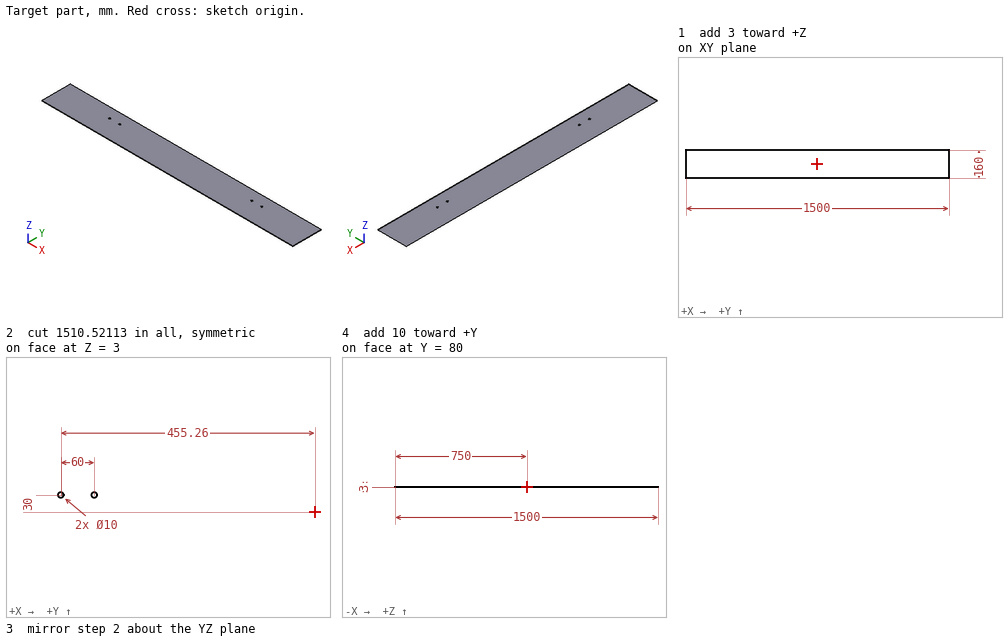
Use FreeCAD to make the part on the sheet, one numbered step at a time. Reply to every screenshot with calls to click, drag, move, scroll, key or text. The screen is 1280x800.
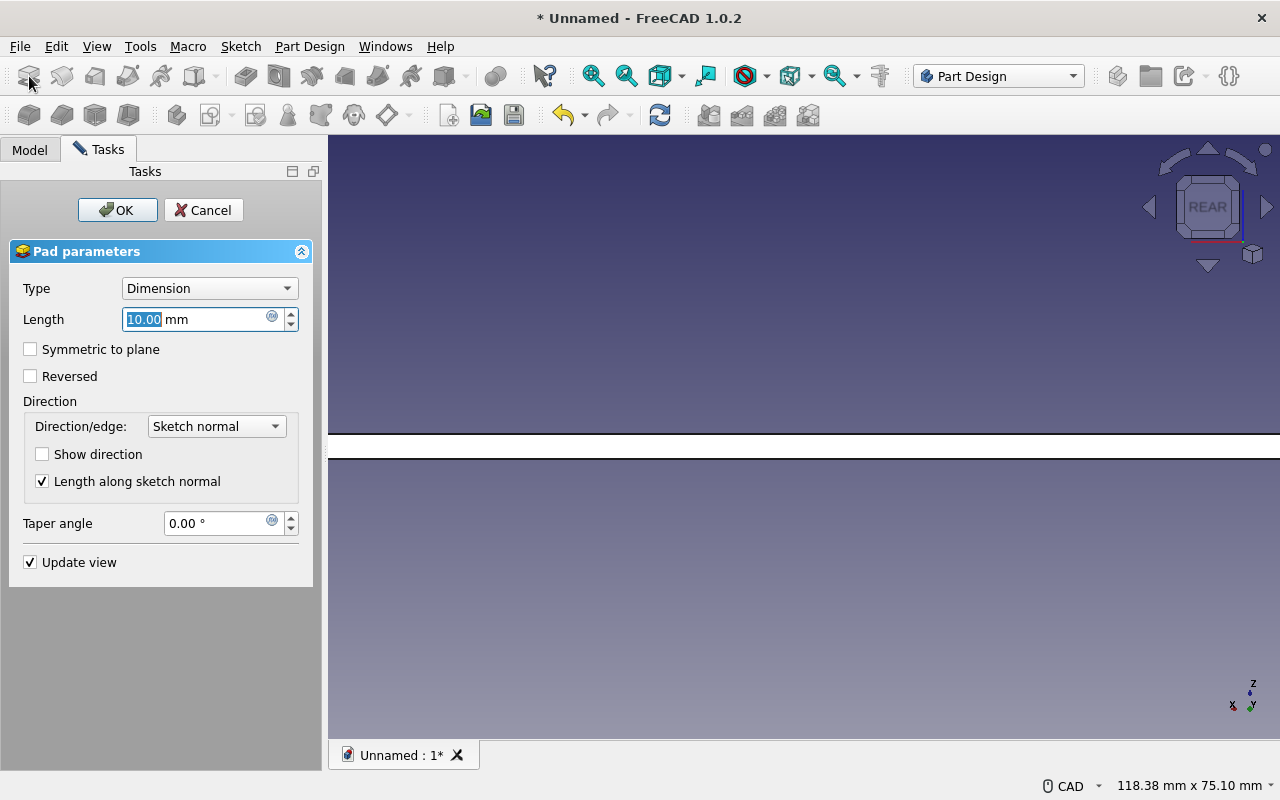
text(10)
key(Tab)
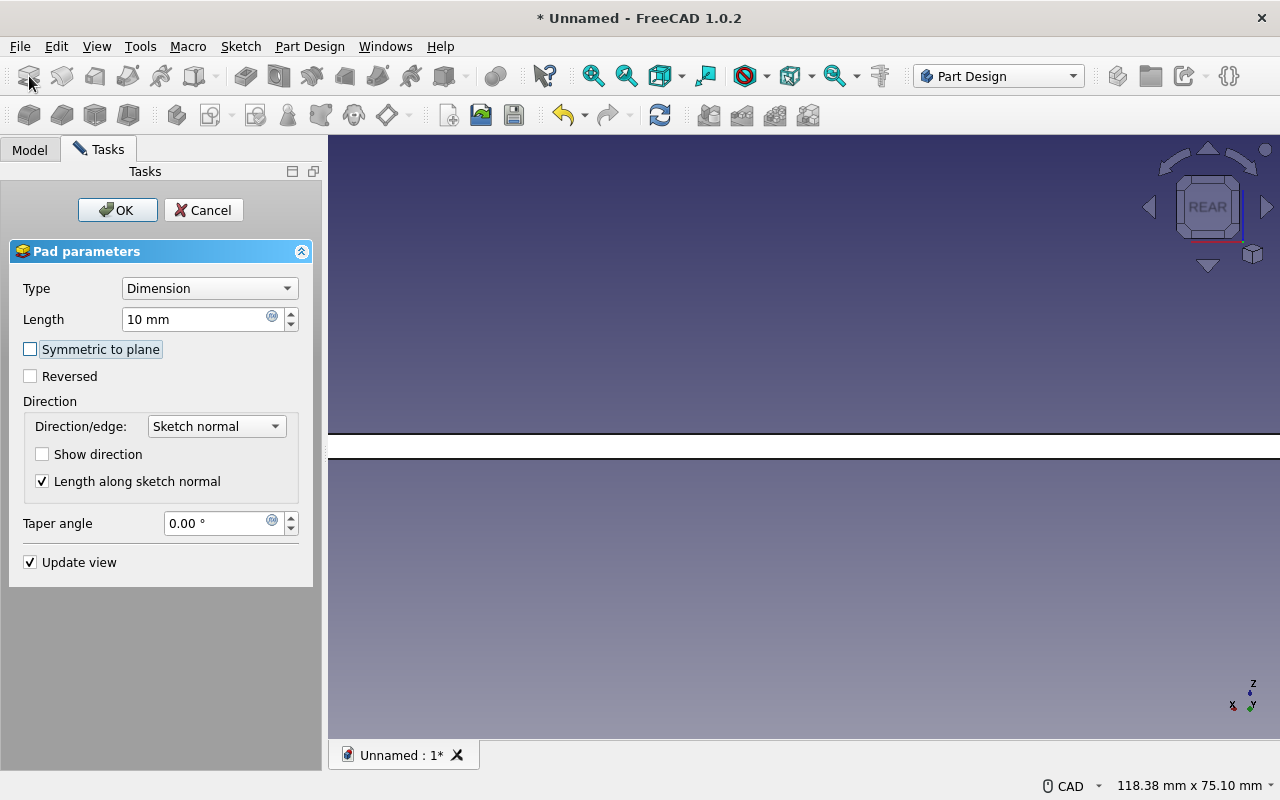
click(118, 210)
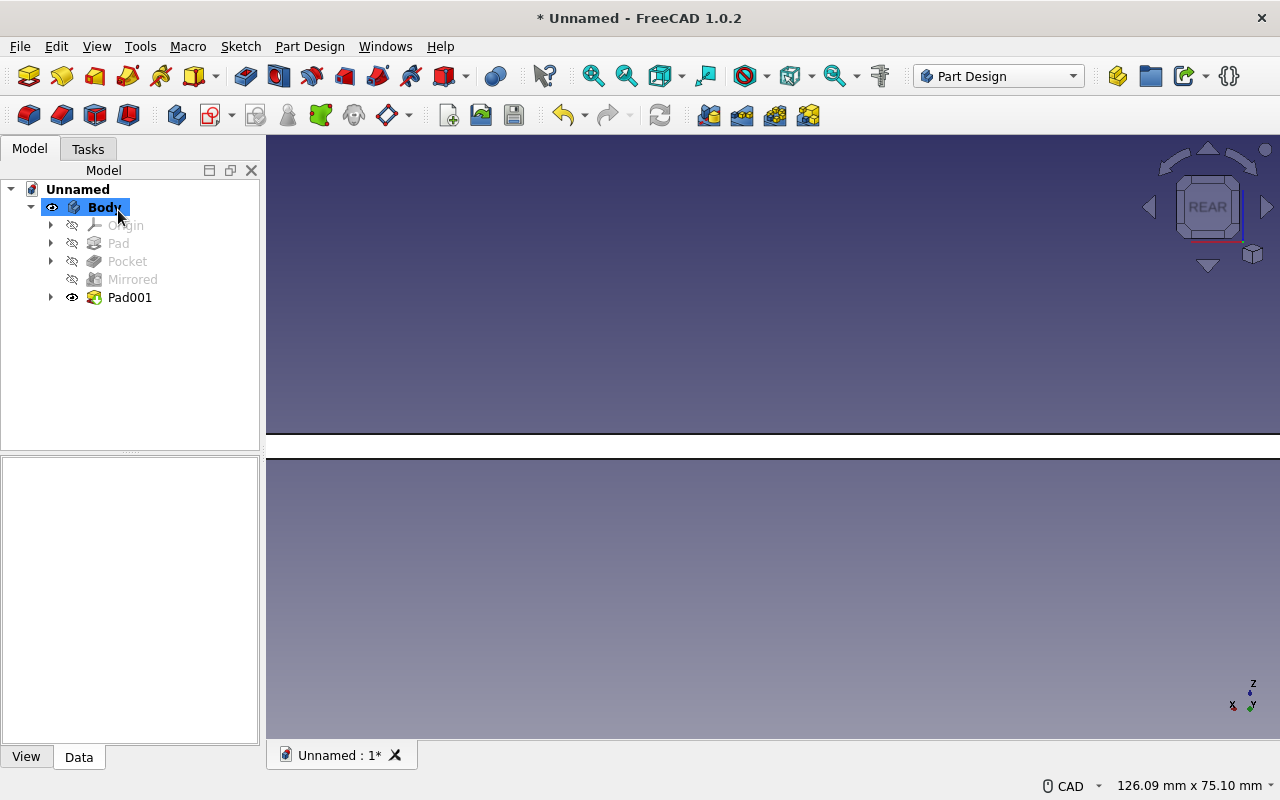
key(0)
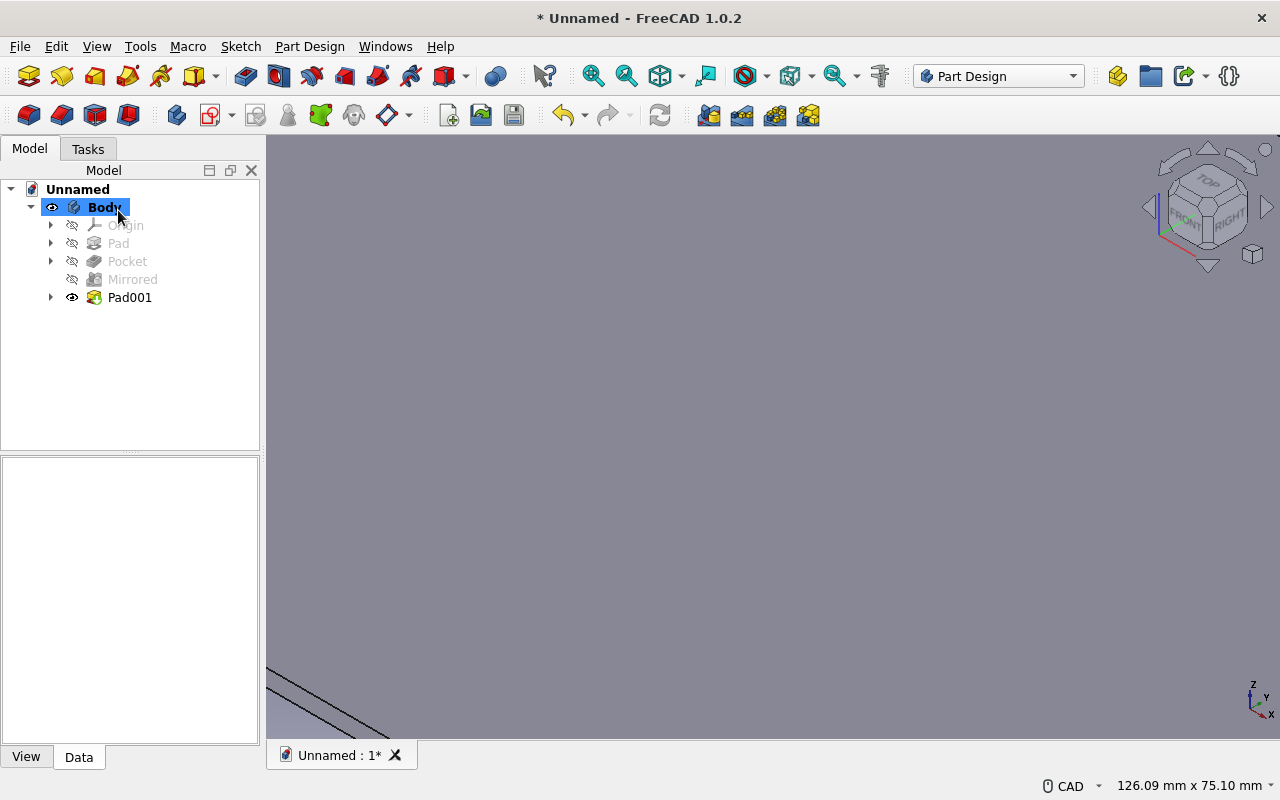
click(594, 76)